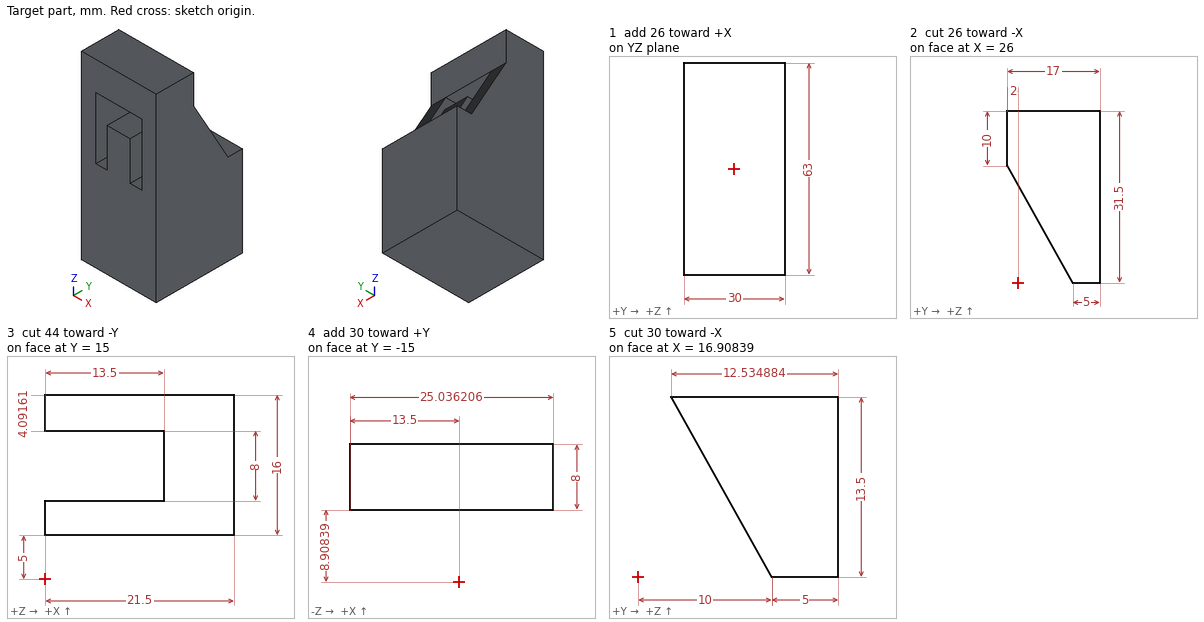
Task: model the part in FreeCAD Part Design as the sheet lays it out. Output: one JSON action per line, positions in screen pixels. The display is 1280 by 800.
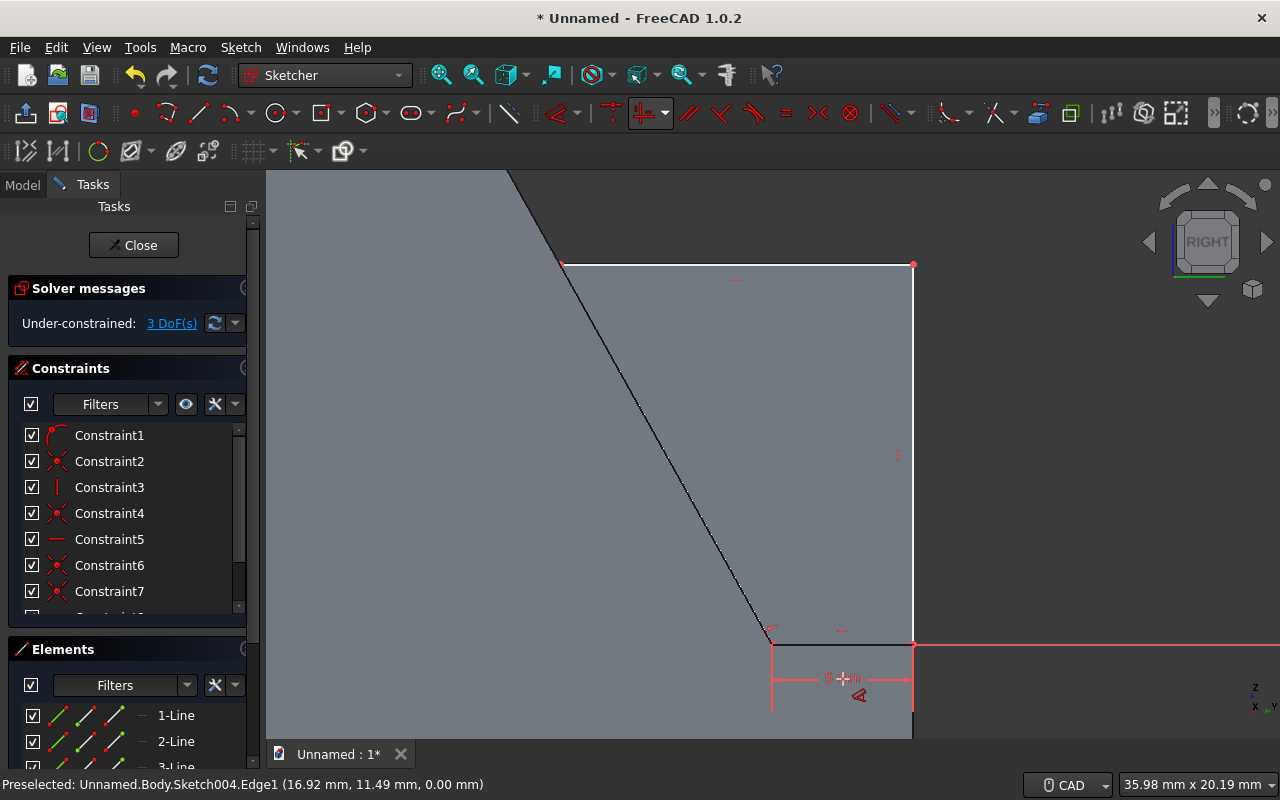
{"action": "left_click", "coordinate": [772, 645]}
{"action": "left_click", "coordinate": [631, 679]}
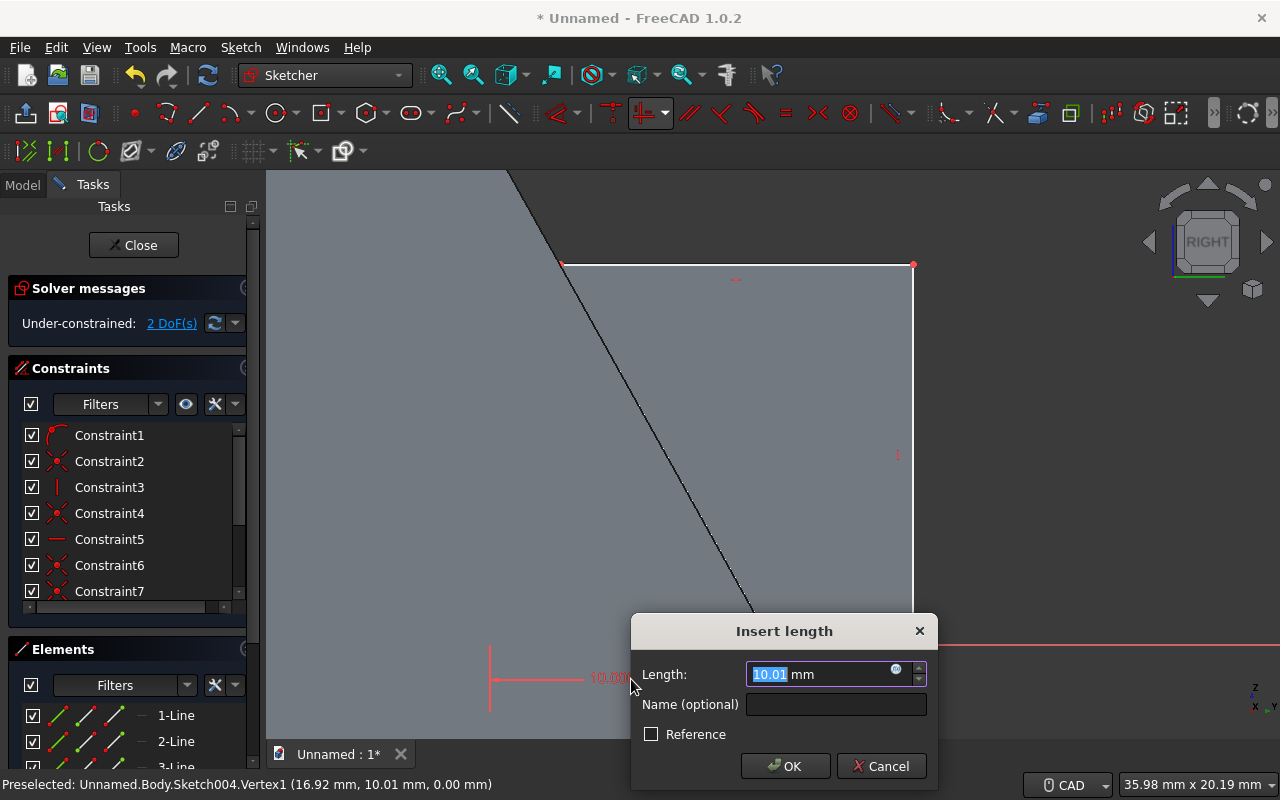
{"action": "type", "text": "10"}
{"action": "key", "text": "Return"}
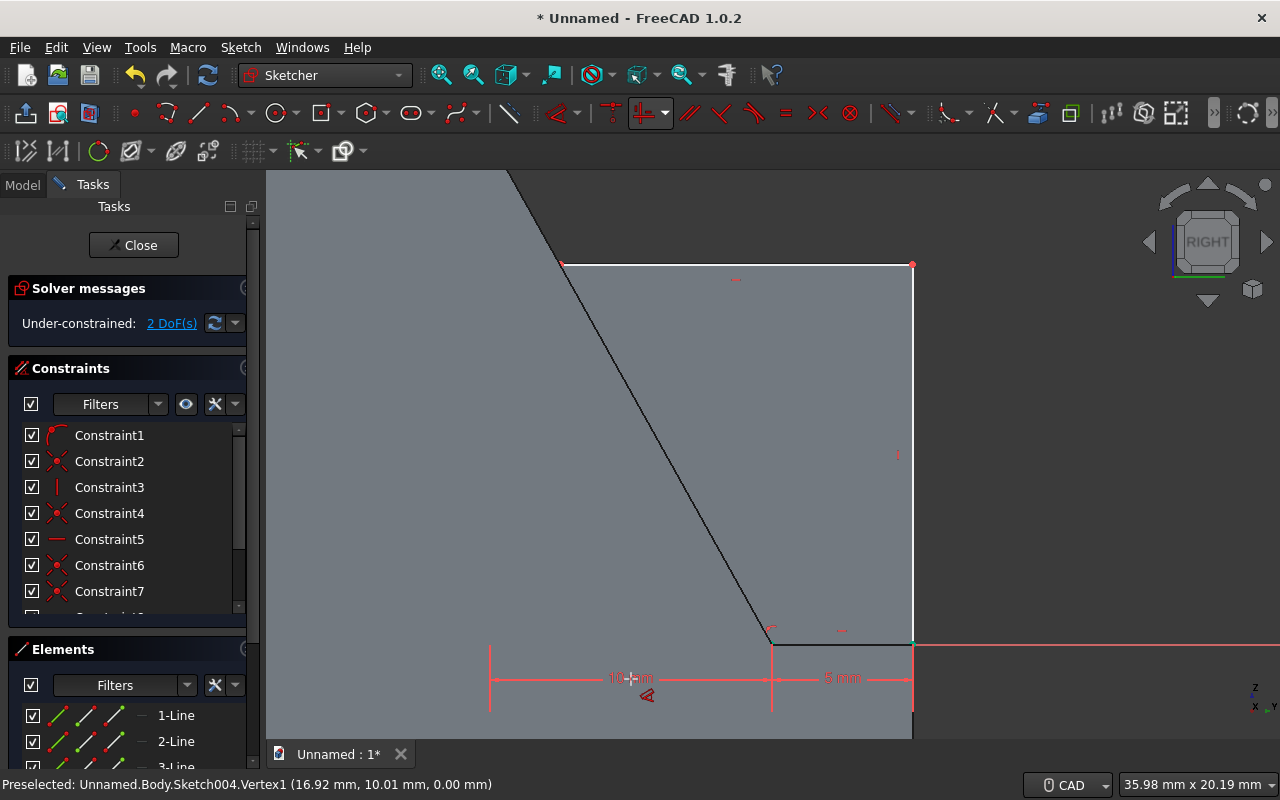
{"action": "left_click", "coordinate": [913, 531]}
{"action": "left_click", "coordinate": [947, 455]}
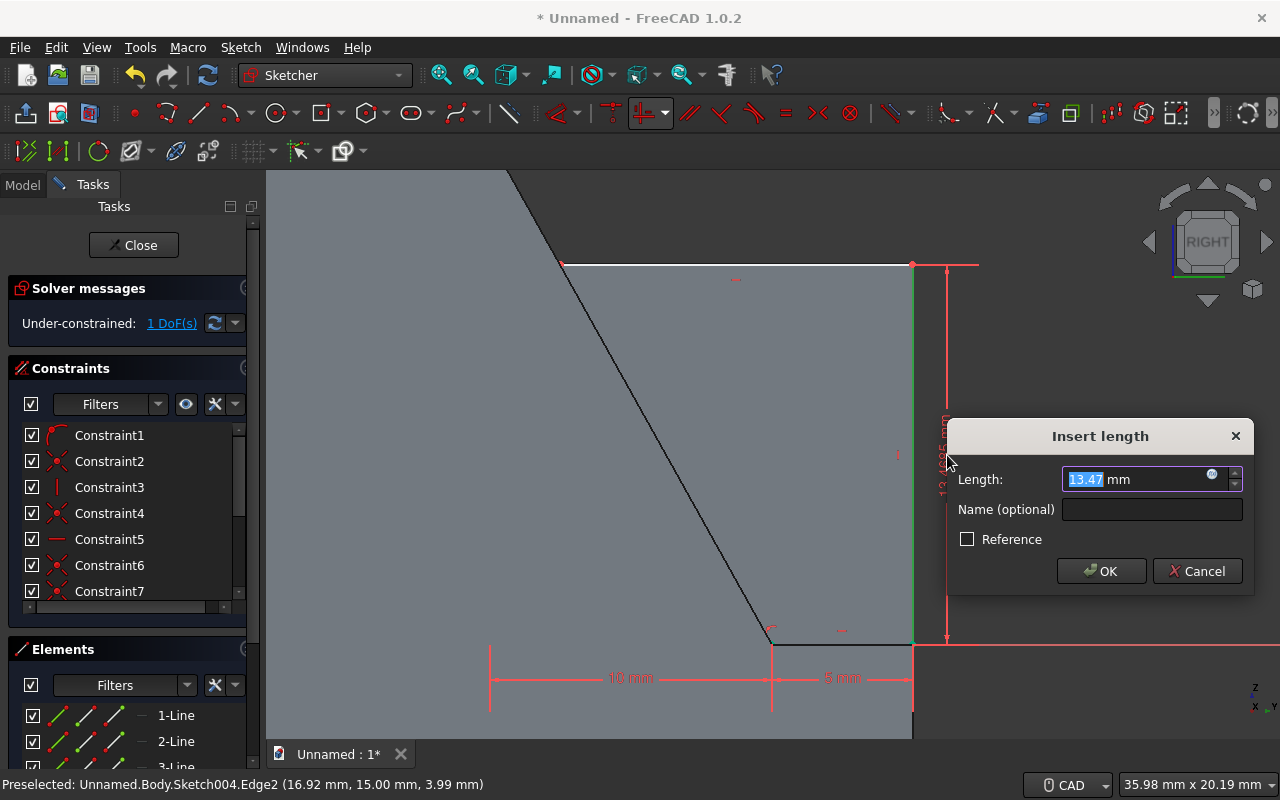
{"action": "type", "text": "13.5"}
{"action": "key", "text": "Return"}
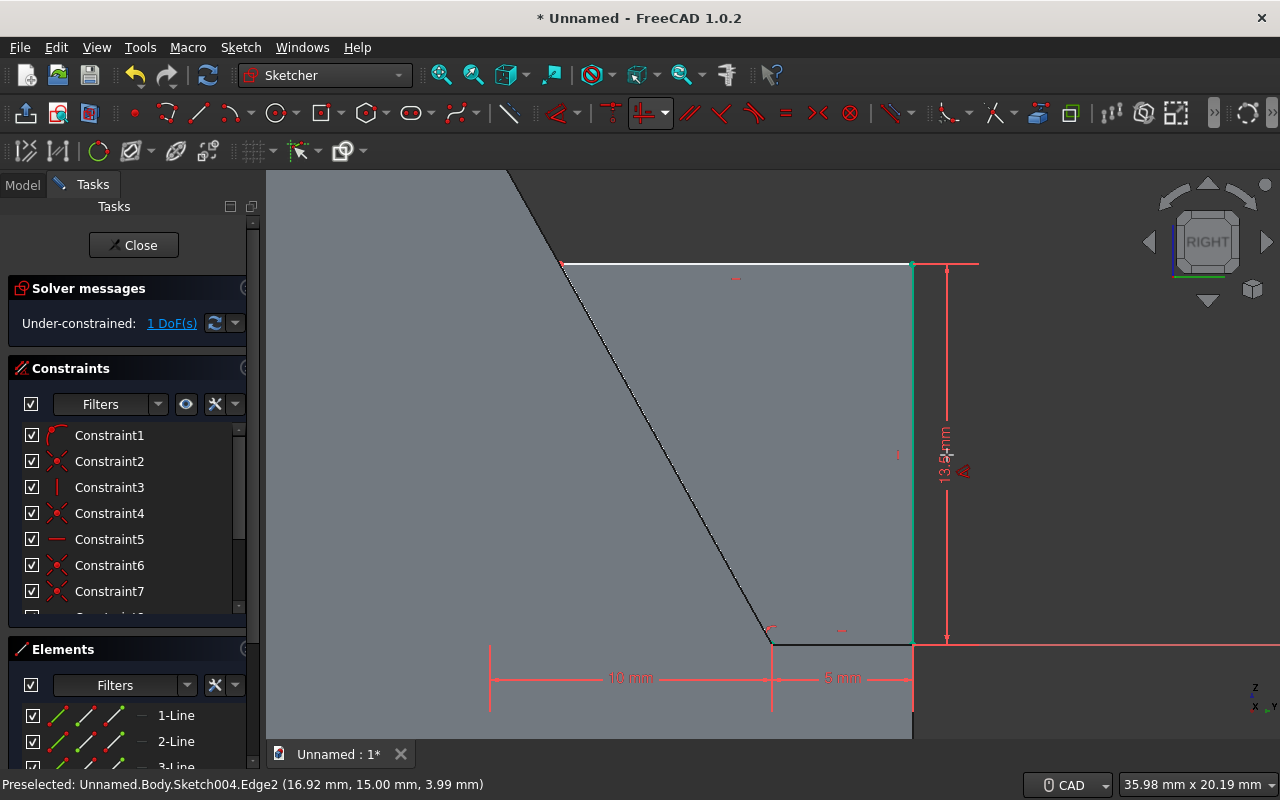
{"action": "left_click", "coordinate": [807, 264]}
{"action": "left_click", "coordinate": [736, 230]}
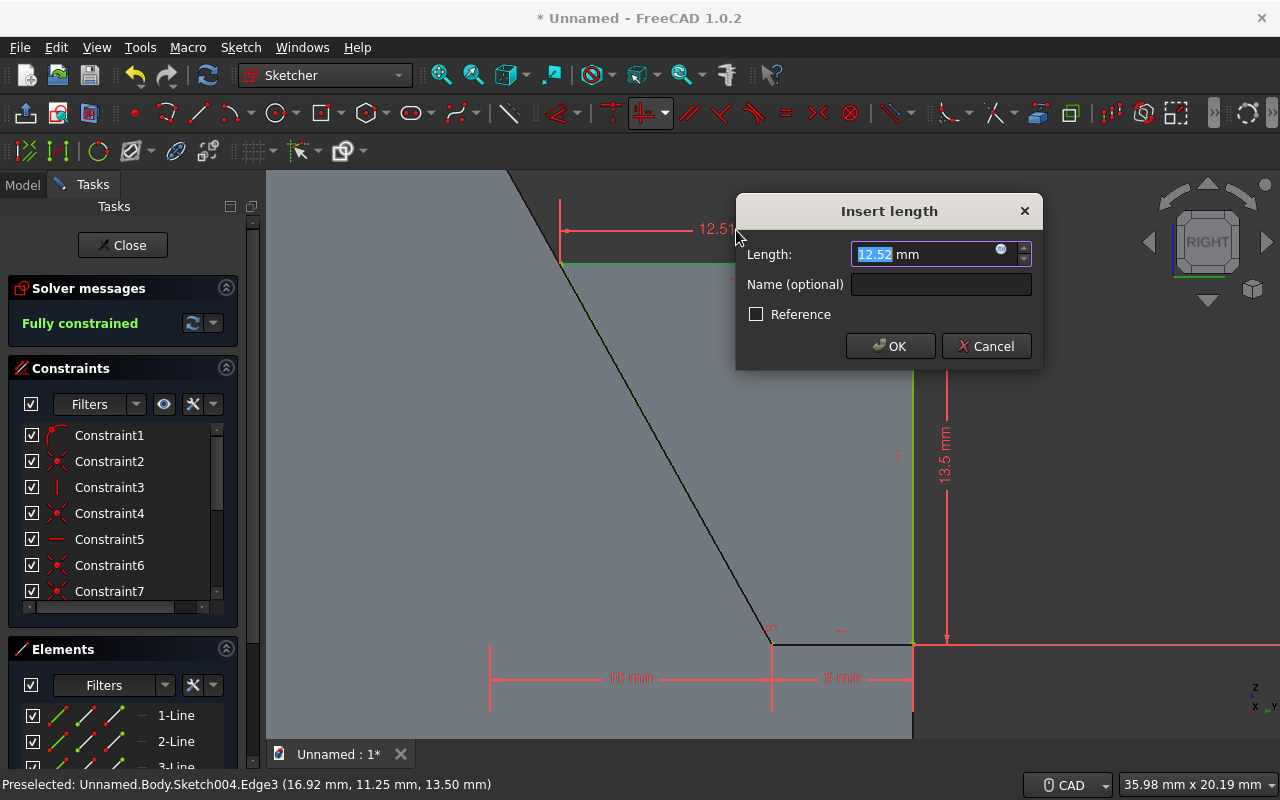
{"action": "type", "text": "12.534884"}
{"action": "key", "text": "Return"}
{"action": "key", "text": "Escape"}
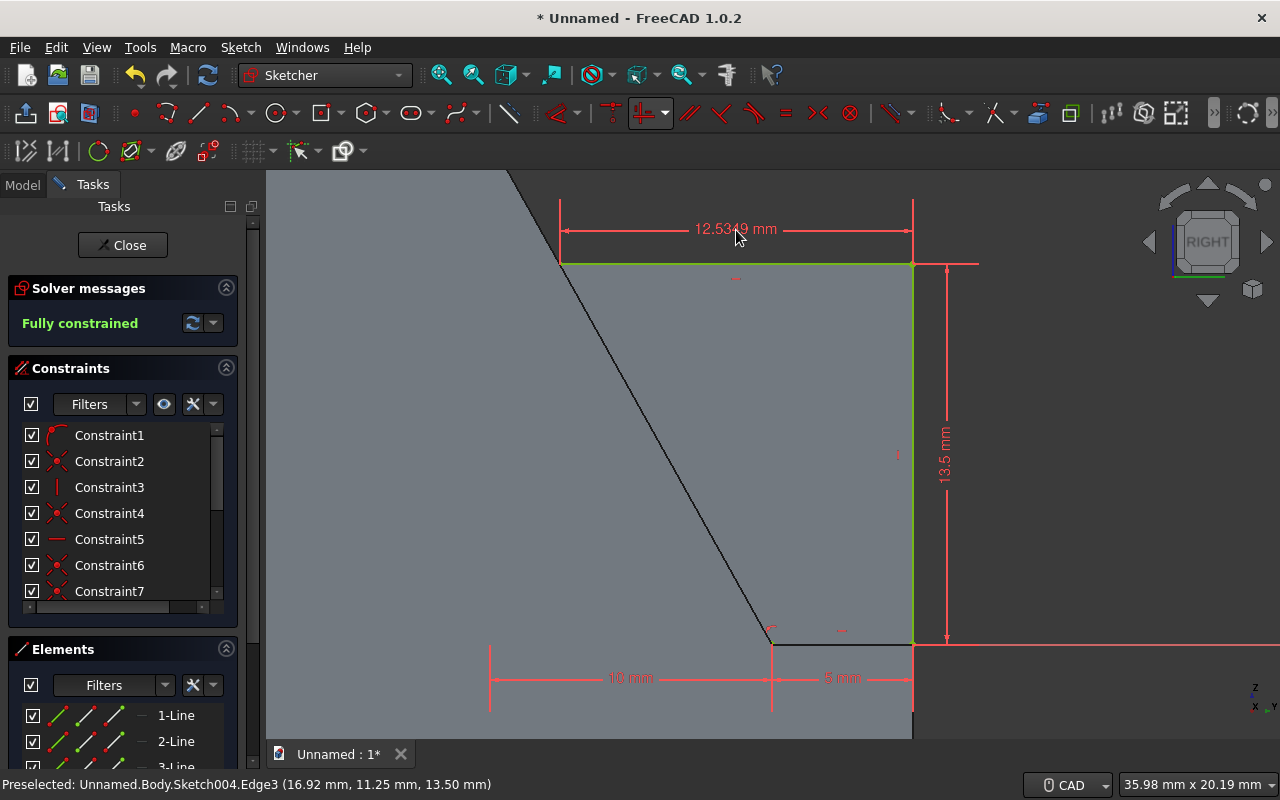
{"action": "left_click", "coordinate": [123, 245]}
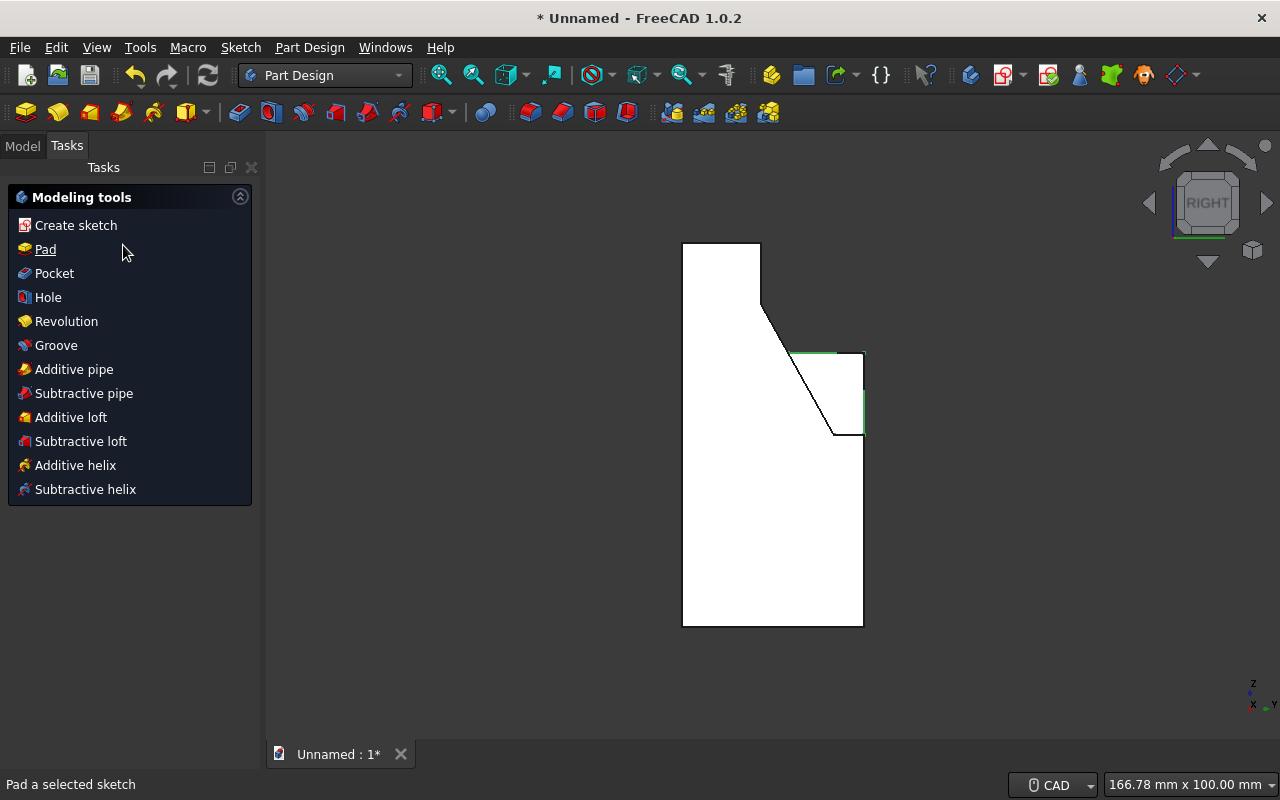
{"action": "left_click", "coordinate": [240, 112]}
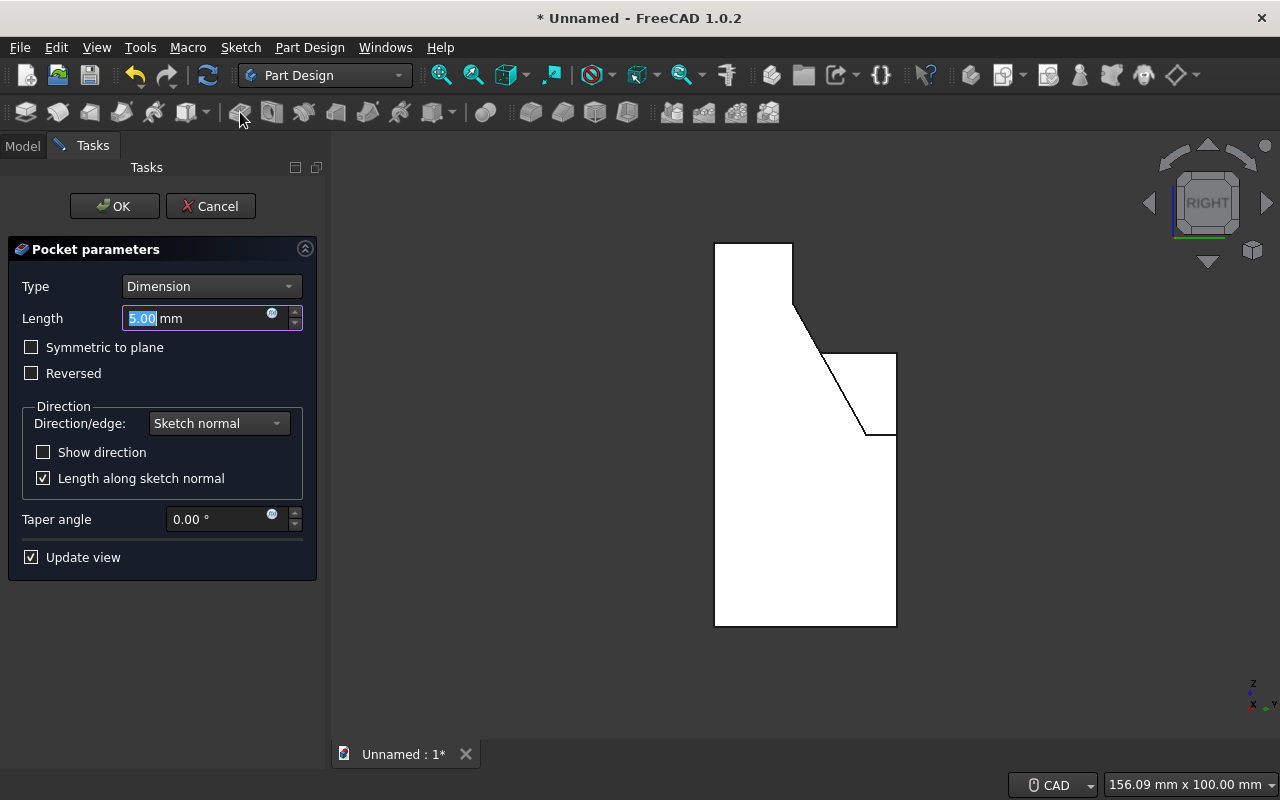
{"action": "type", "text": "30"}
{"action": "key", "text": "Tab"}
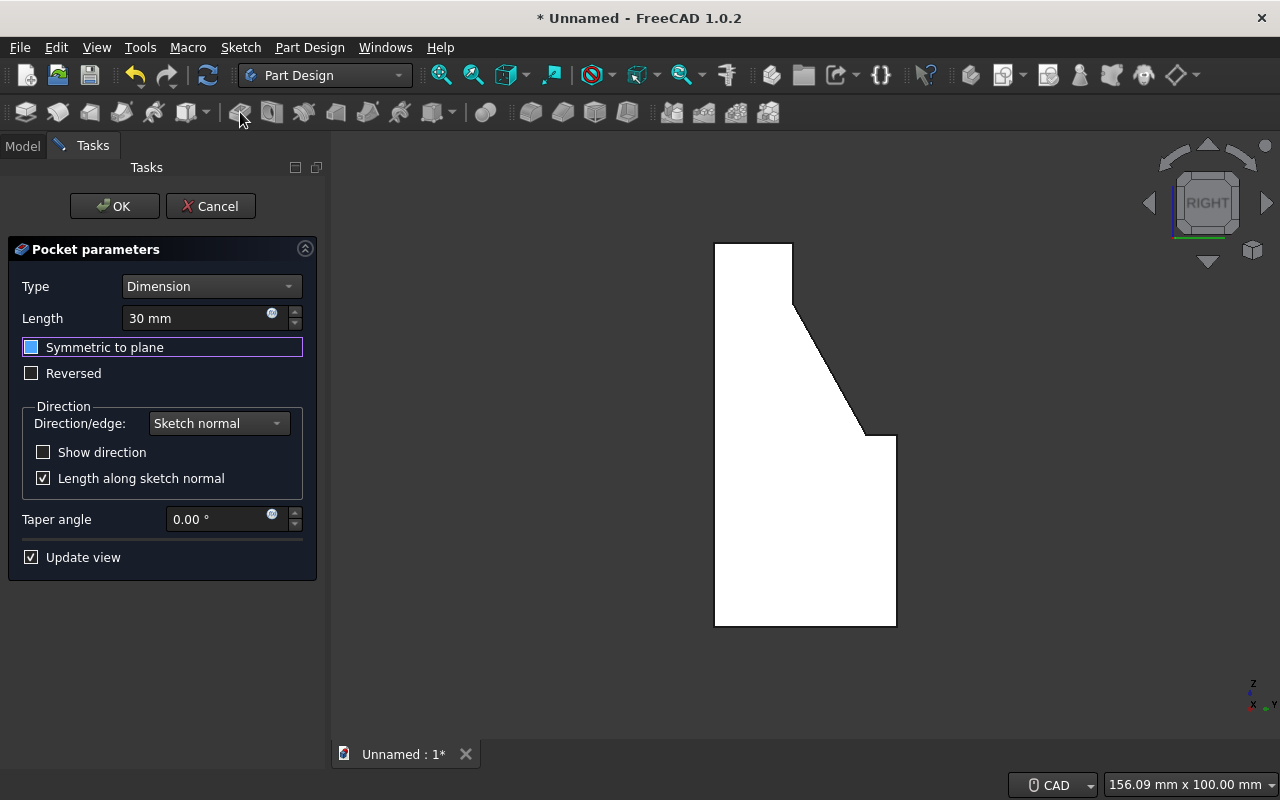
{"action": "left_click", "coordinate": [115, 206]}